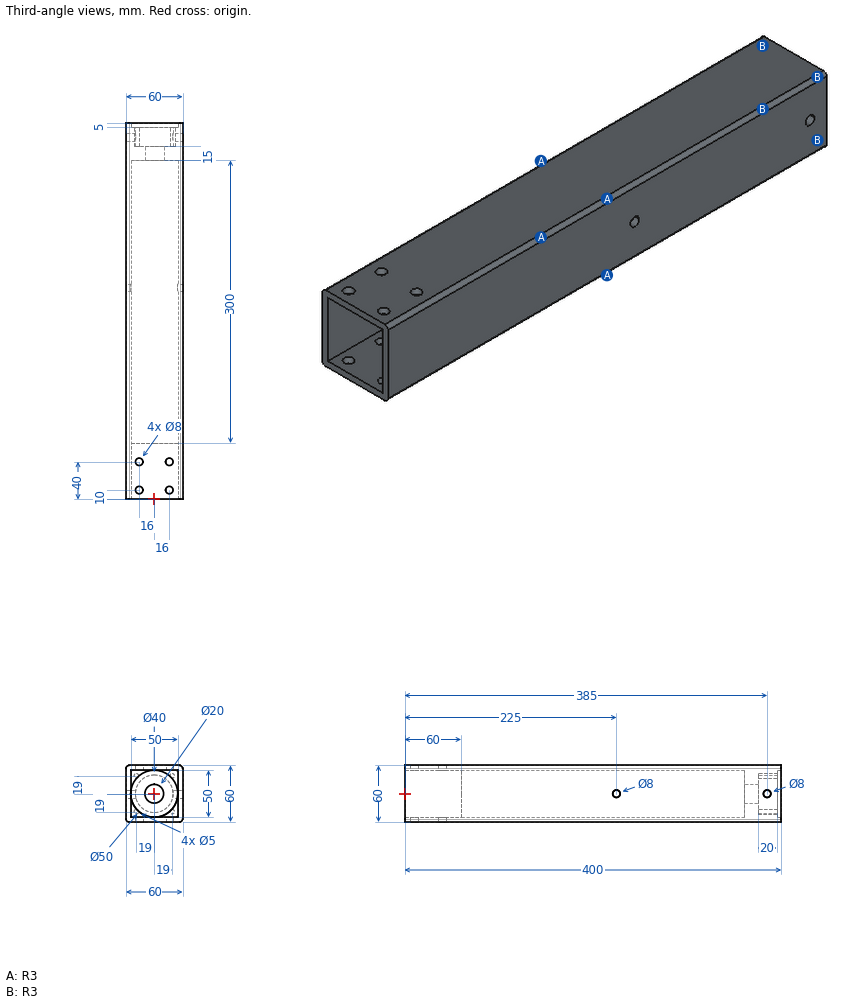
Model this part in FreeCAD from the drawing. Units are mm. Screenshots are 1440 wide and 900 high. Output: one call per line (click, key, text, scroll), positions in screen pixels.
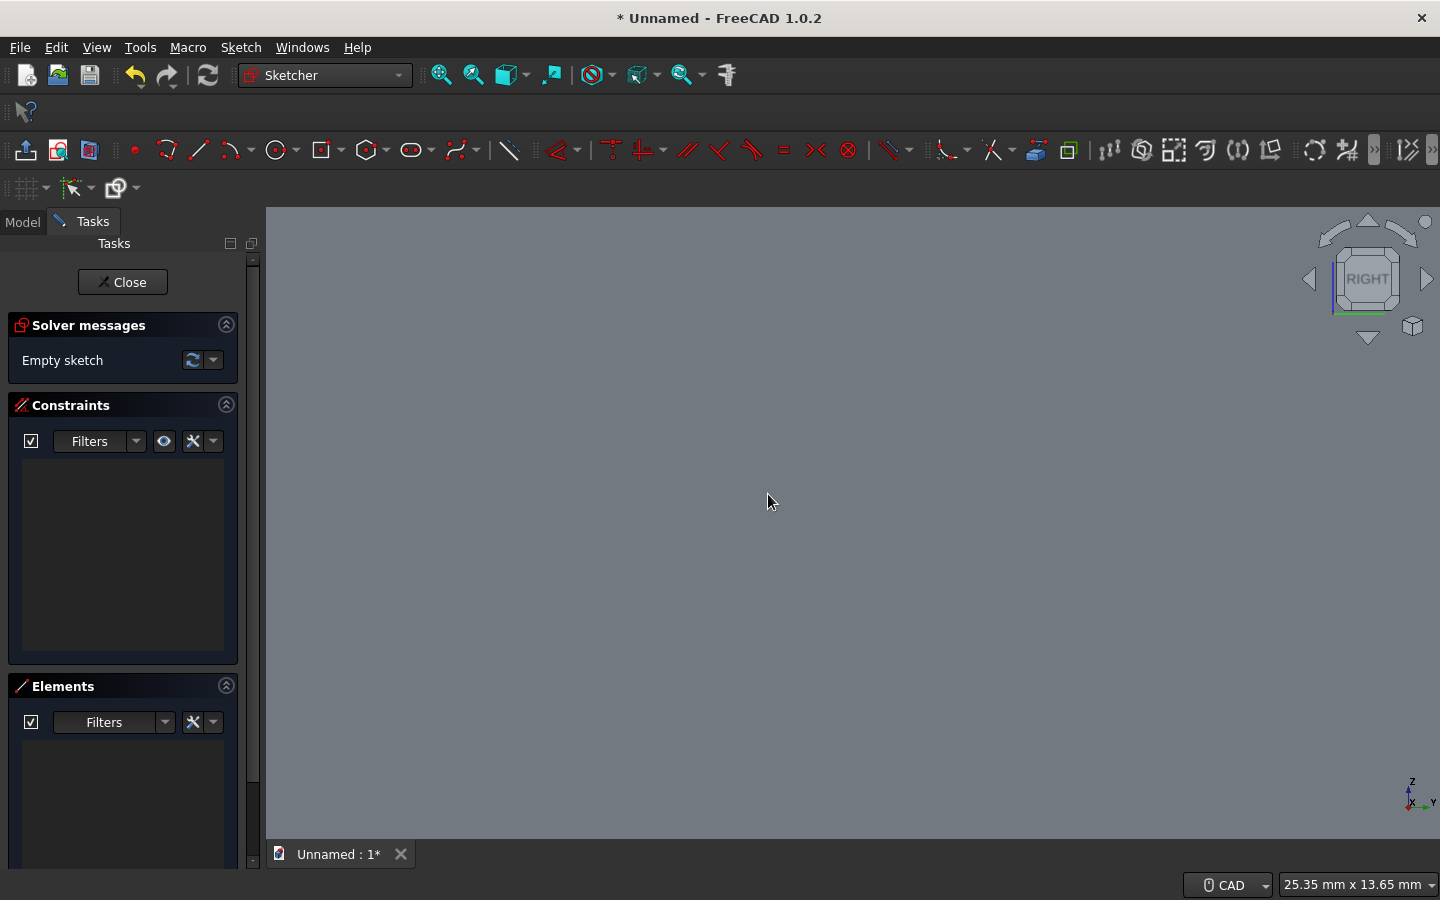
key(g)
key(c)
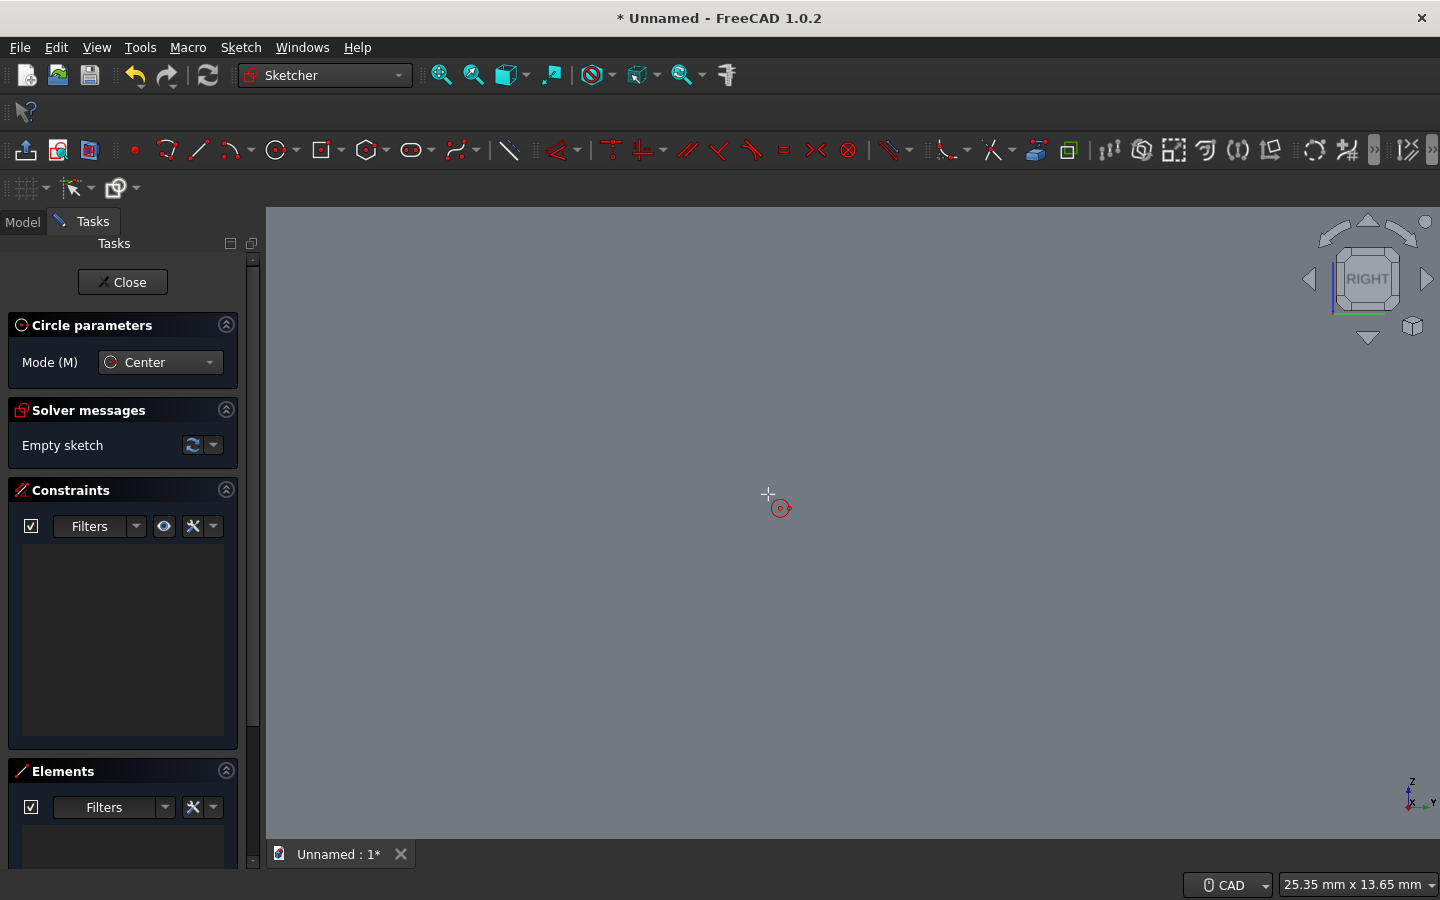
click(784, 523)
move(915, 392)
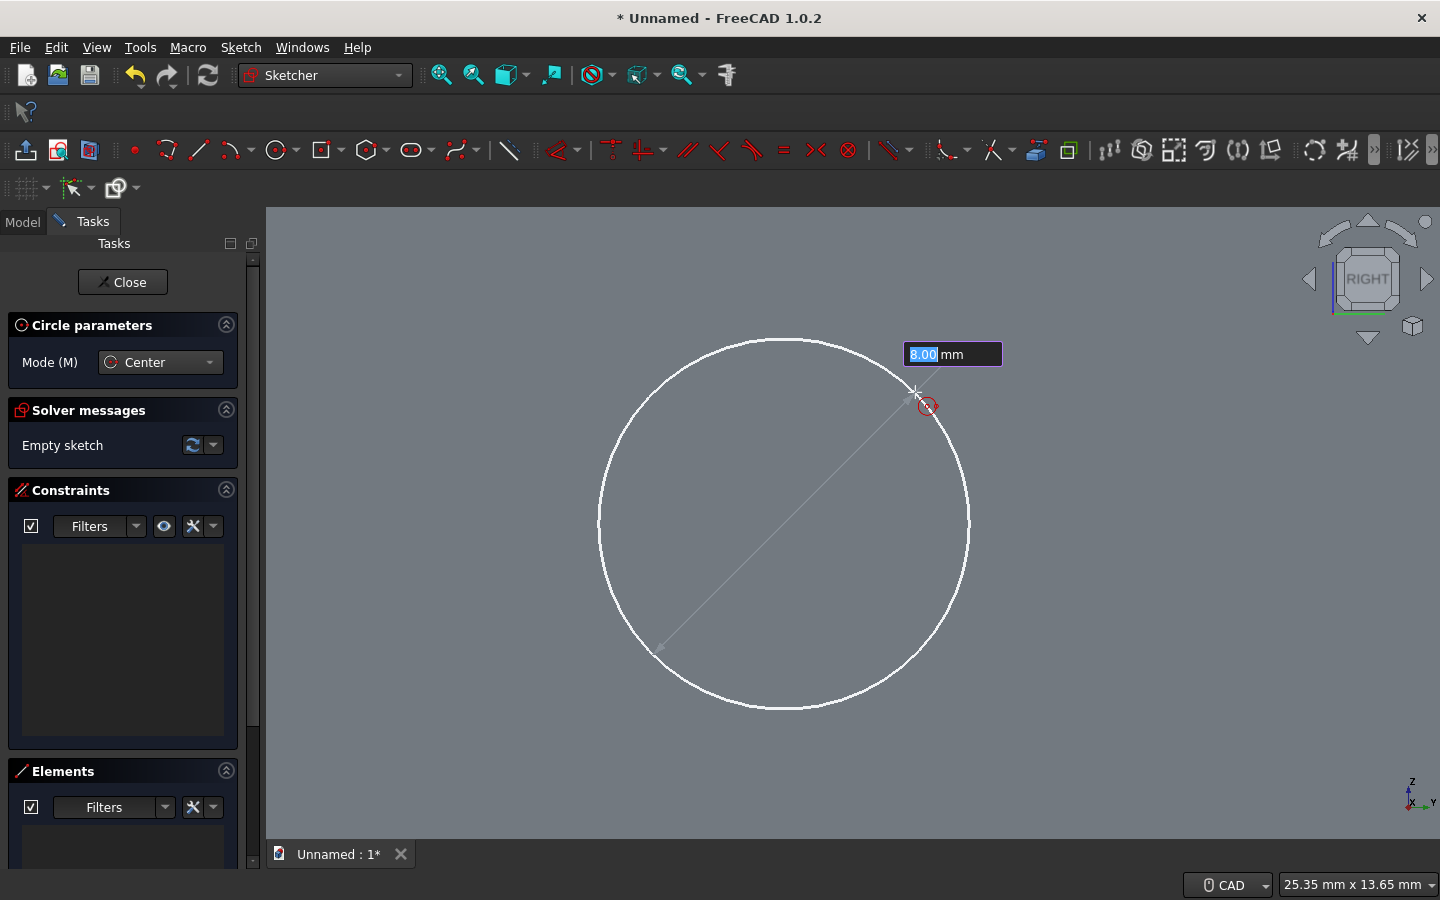
text(8)
key(Return)
key(Escape)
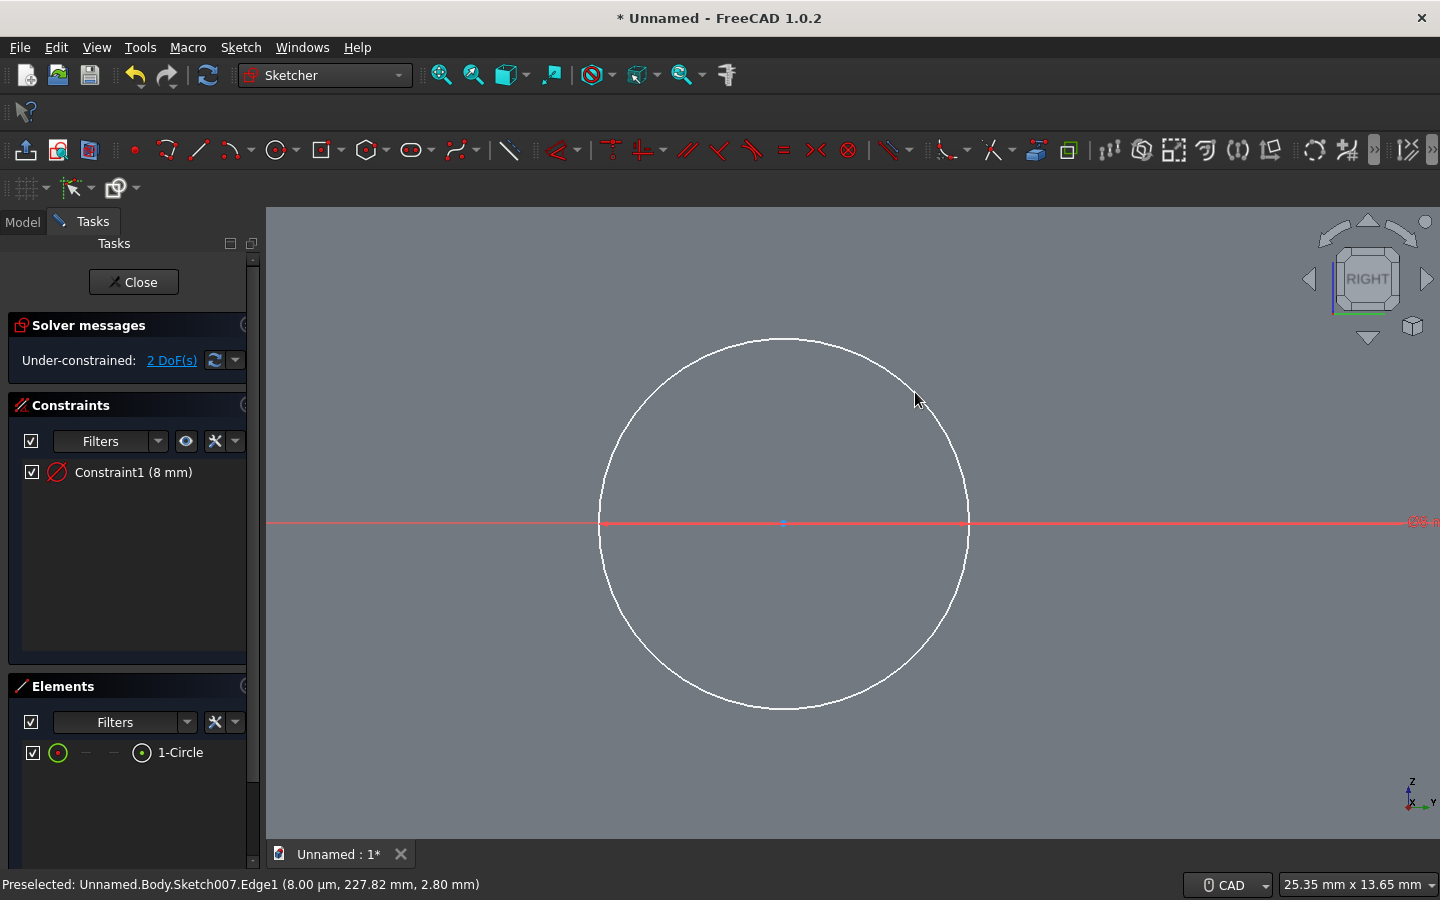
click(784, 524)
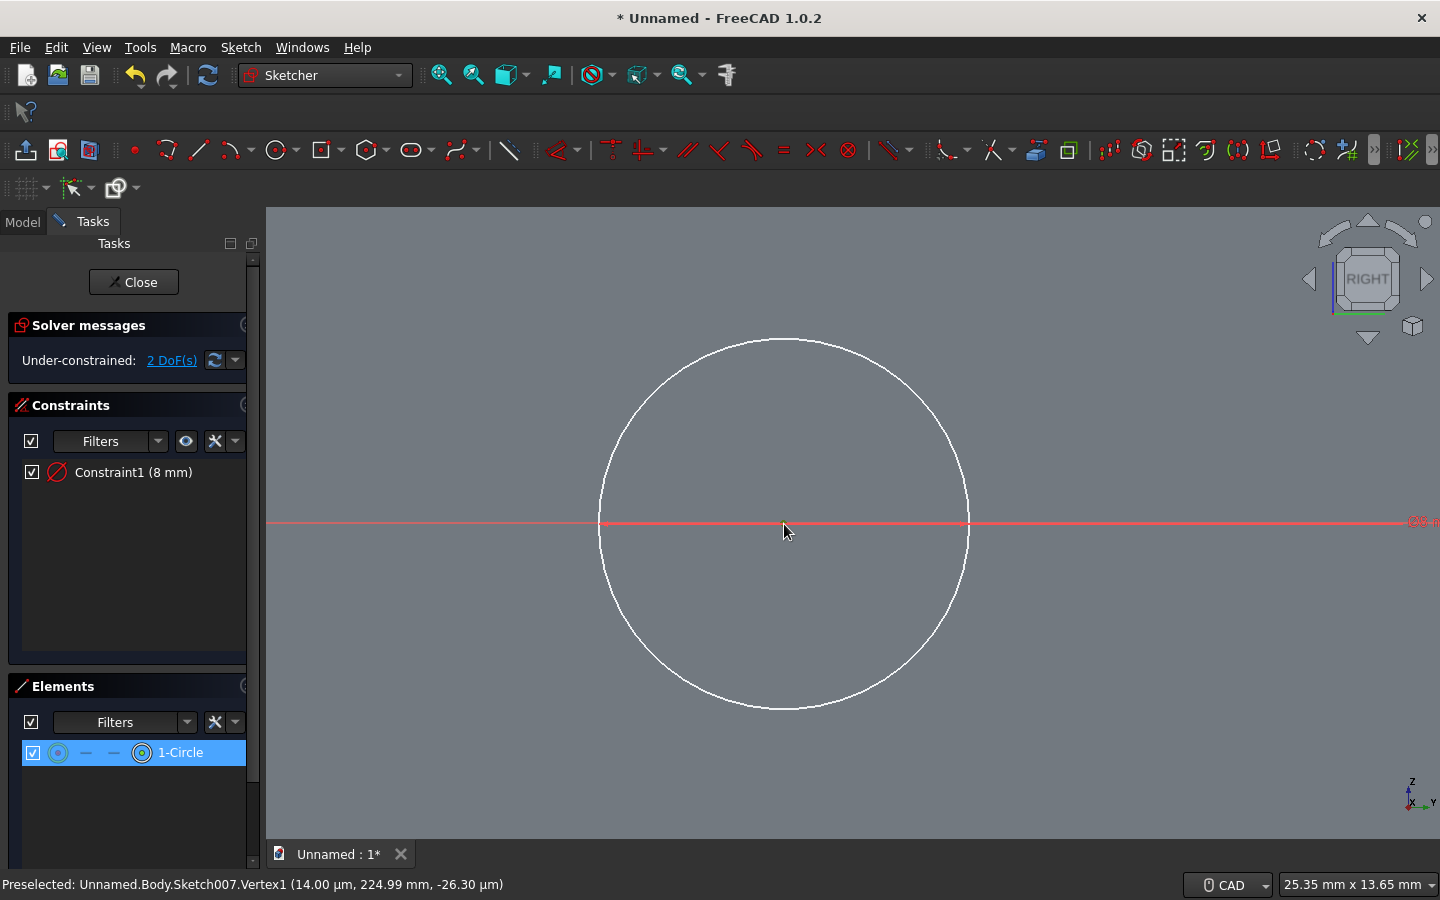
click(364, 523)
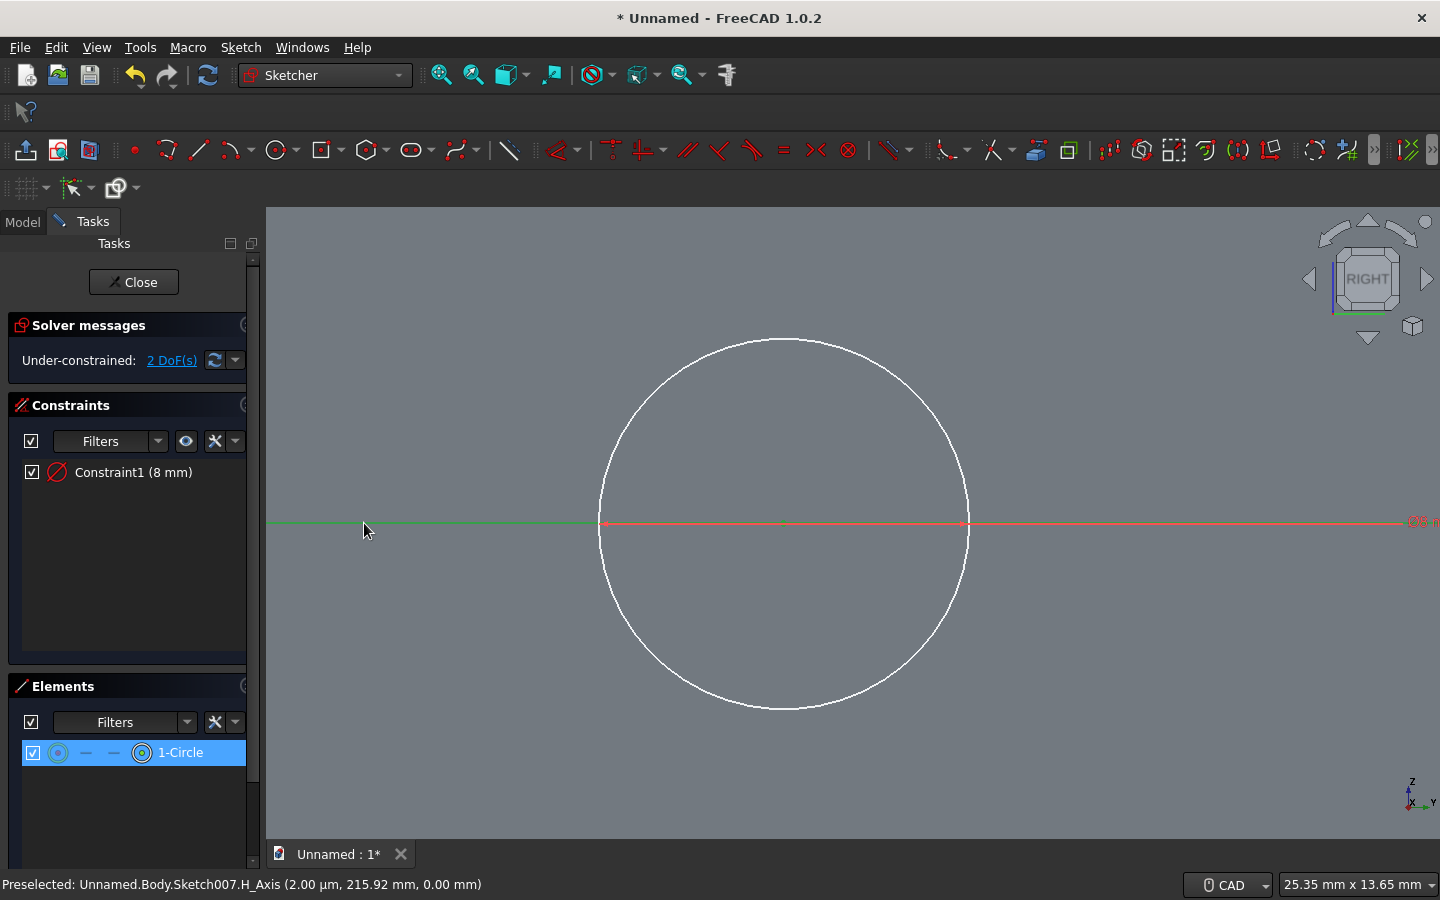
click(612, 150)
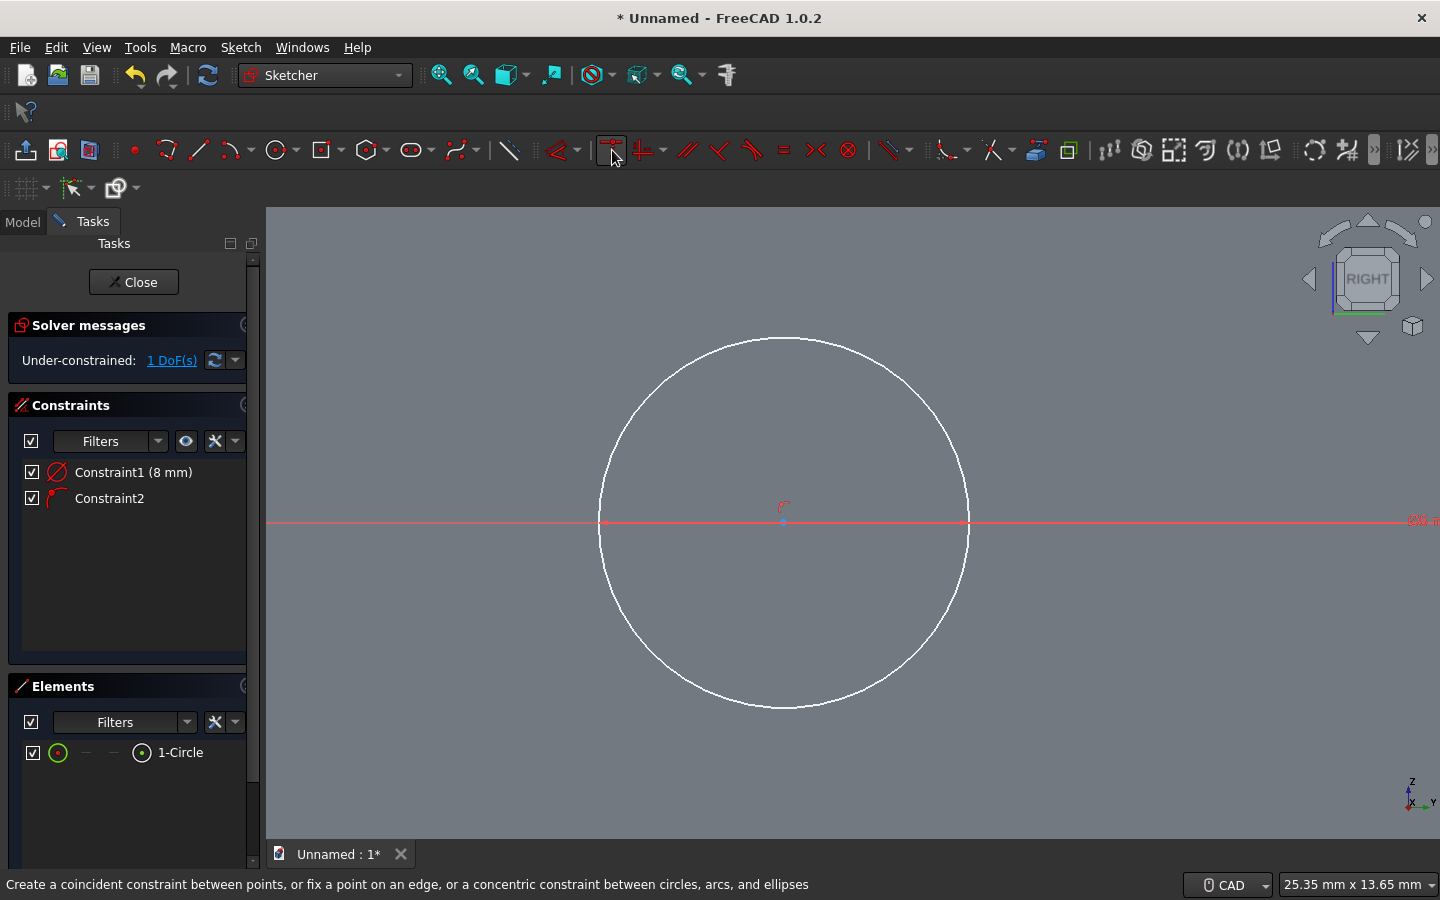
click(556, 150)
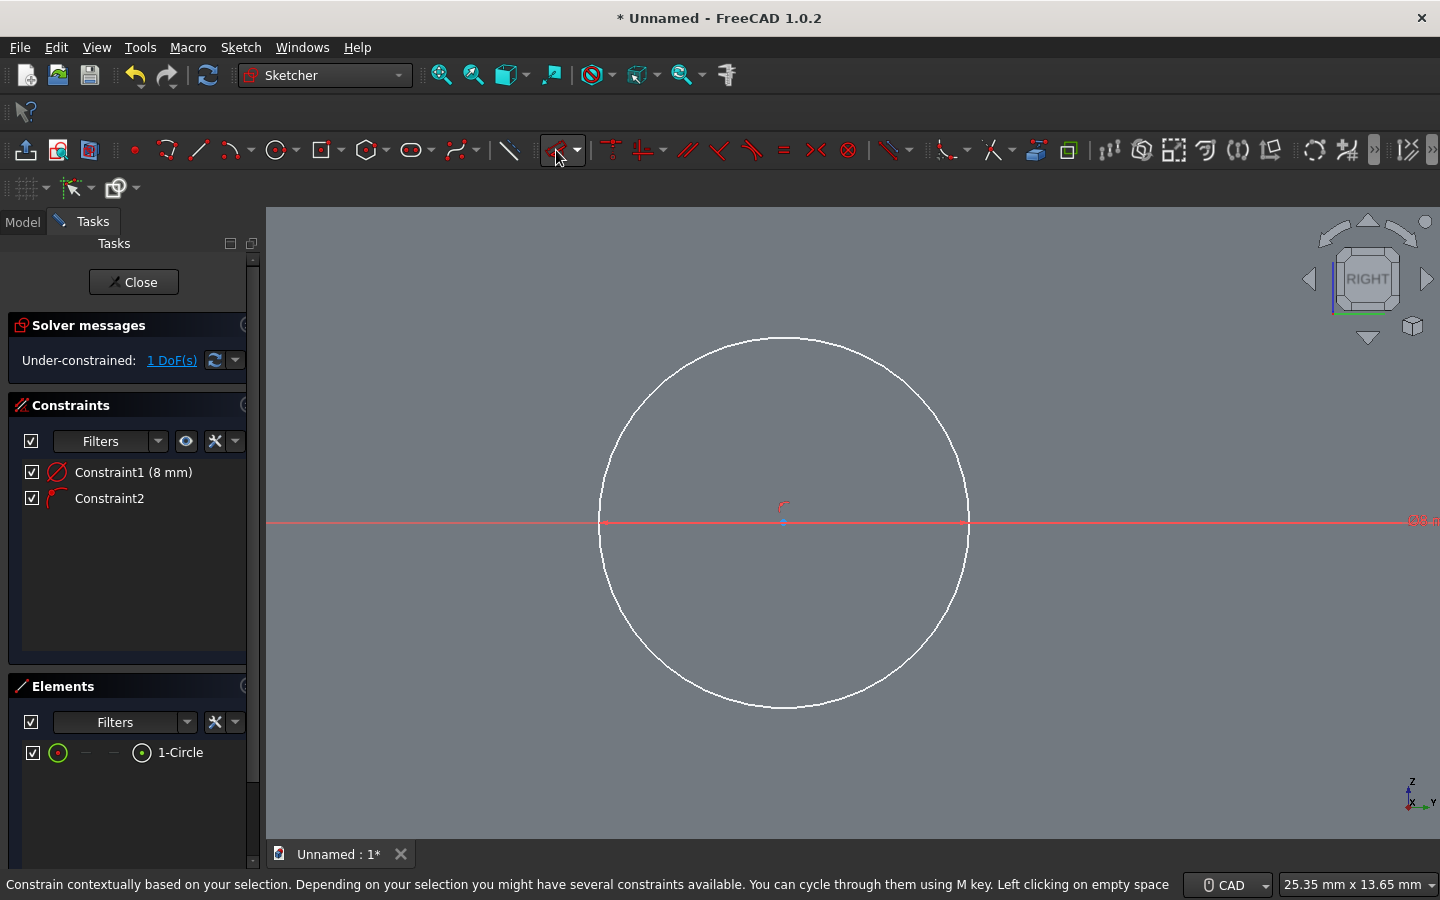
click(784, 523)
click(539, 557)